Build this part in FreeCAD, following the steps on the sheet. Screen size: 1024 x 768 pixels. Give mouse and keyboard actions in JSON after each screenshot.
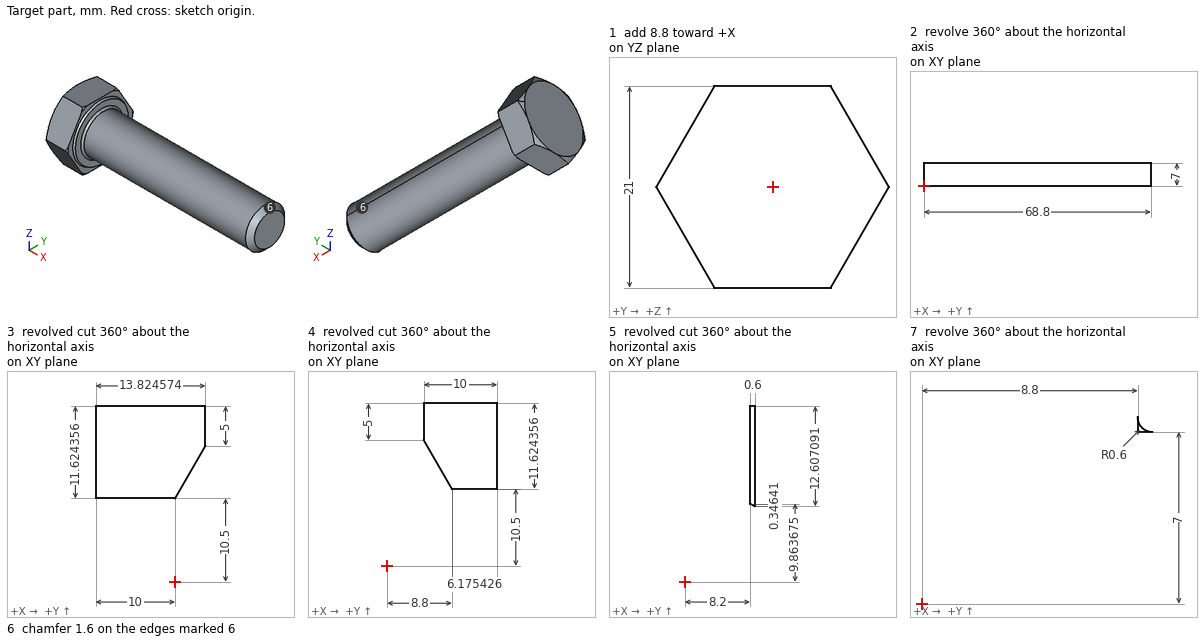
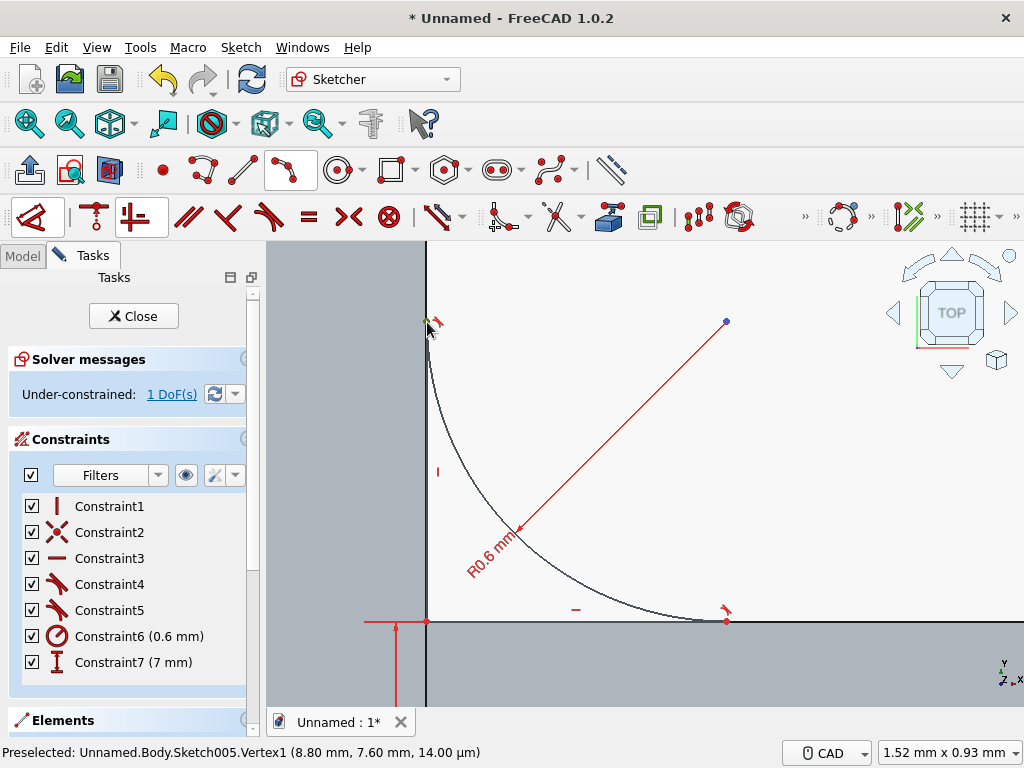
{"action": "key", "text": "l"}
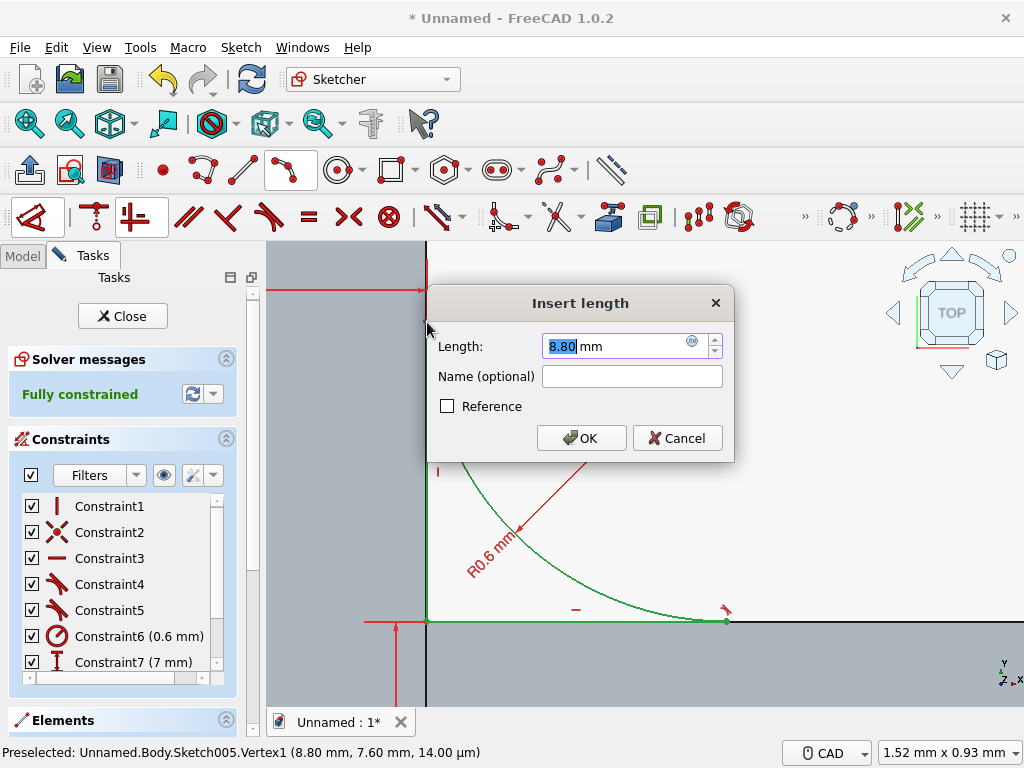
{"action": "type", "text": "8.8"}
{"action": "key", "text": "Return"}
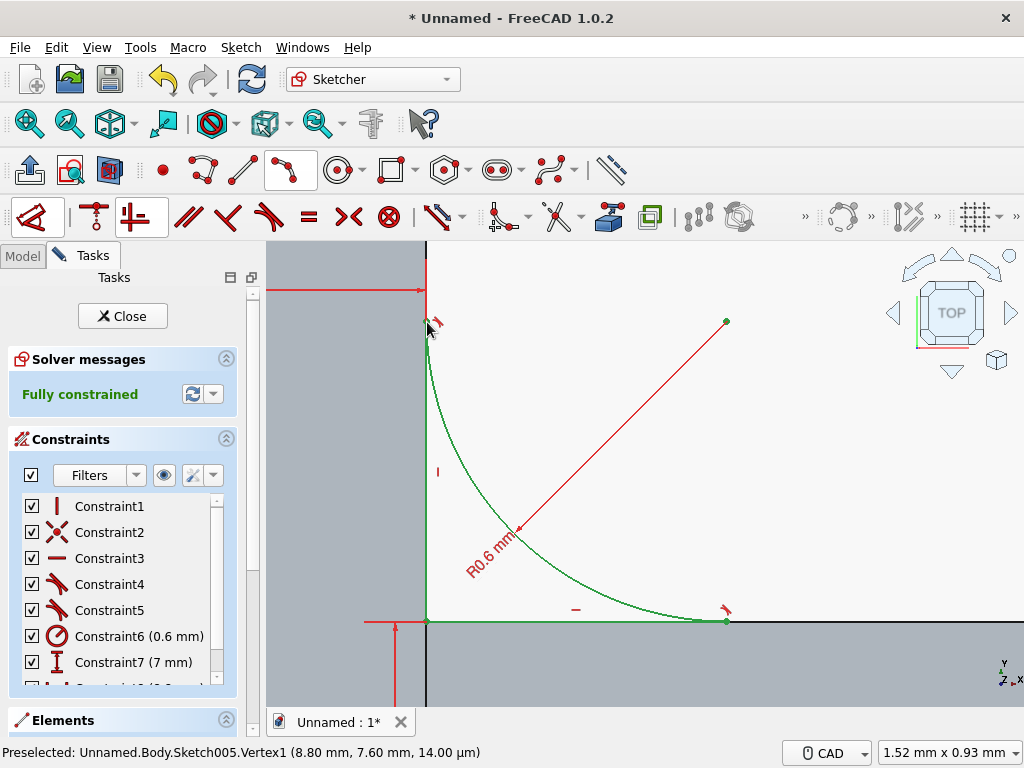
{"action": "left_click", "coordinate": [123, 316]}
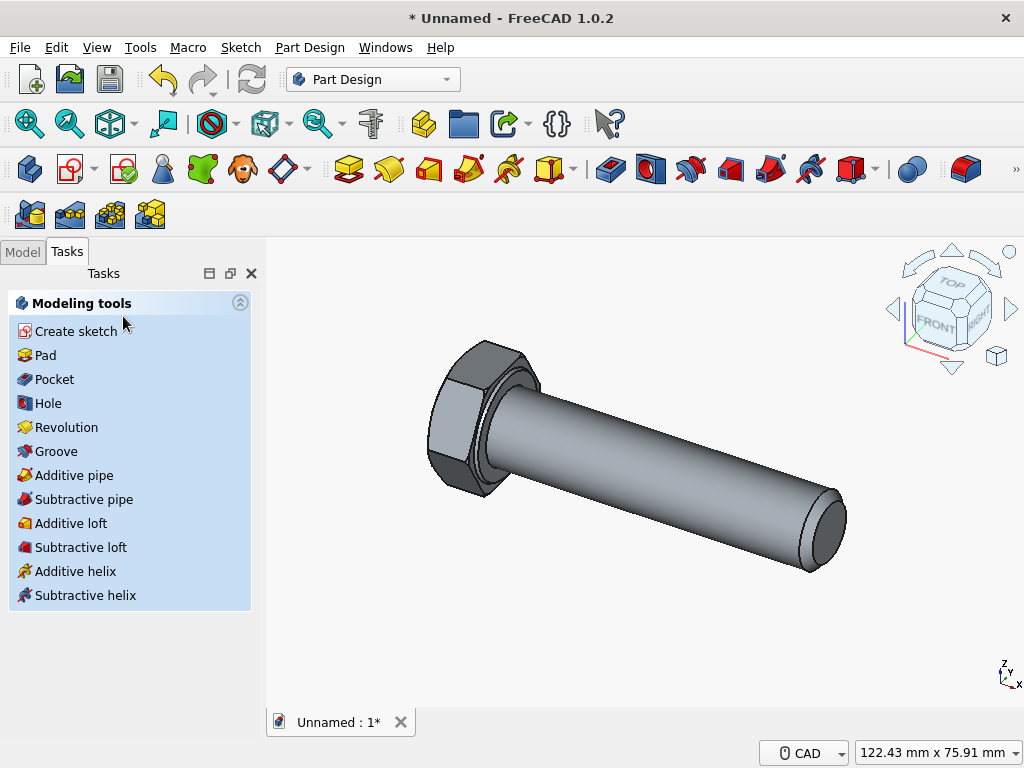
{"action": "left_click", "coordinate": [390, 170]}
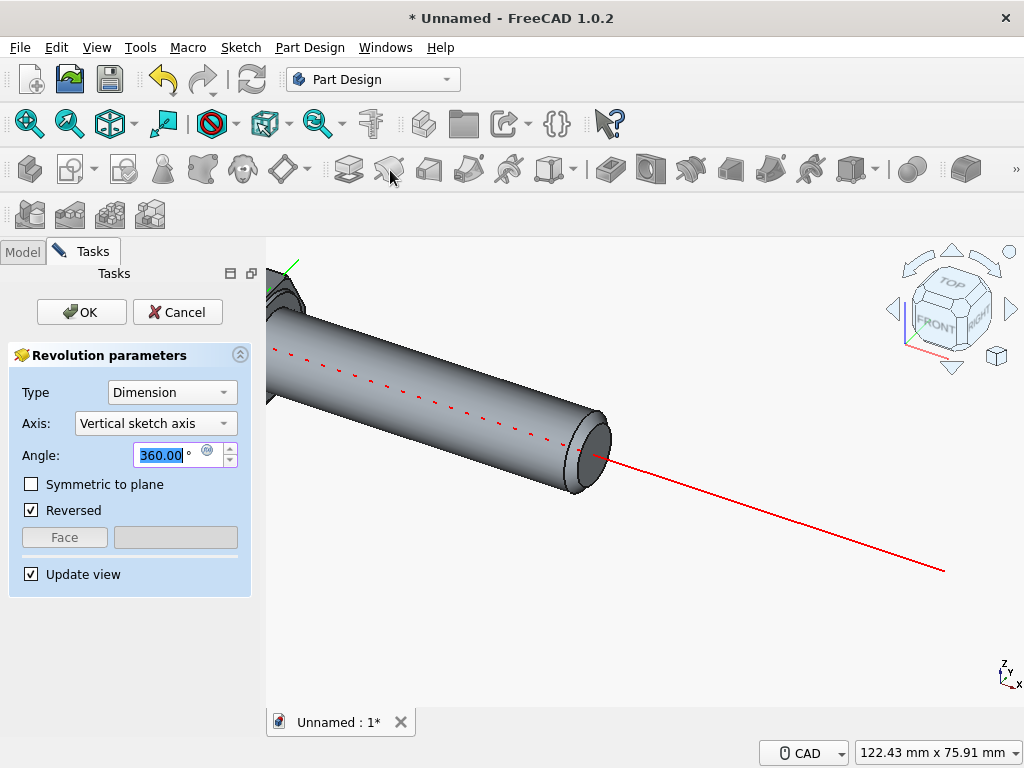
{"action": "left_click", "coordinate": [156, 424]}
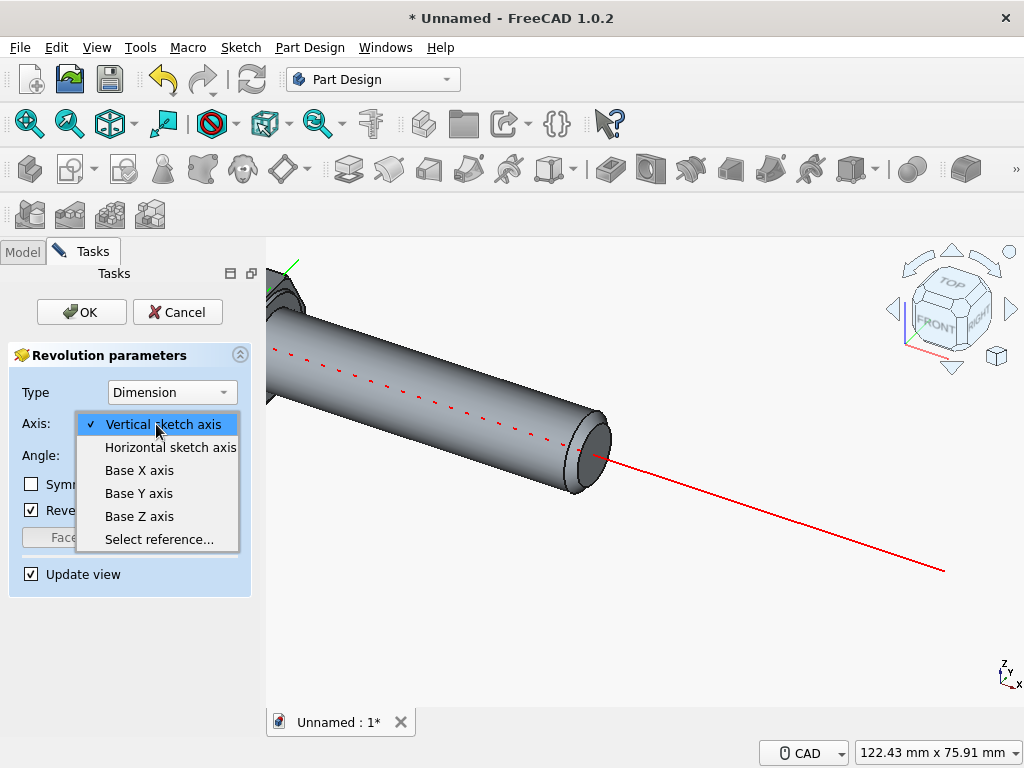
{"action": "left_click", "coordinate": [156, 448]}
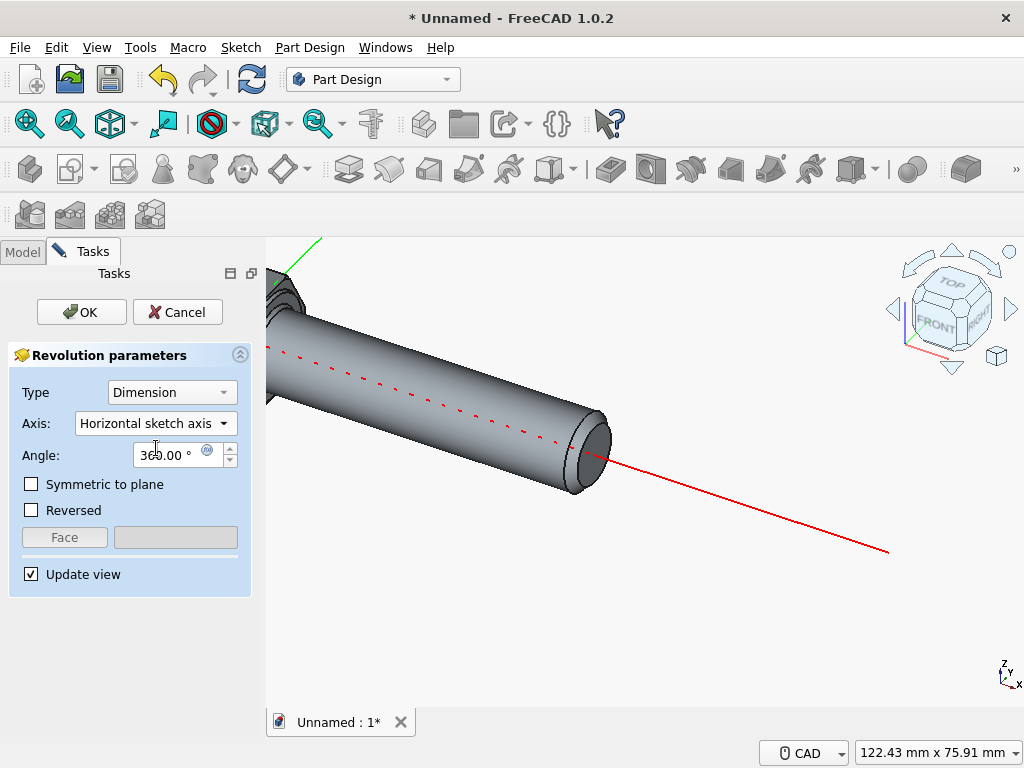
{"action": "left_click", "coordinate": [82, 312]}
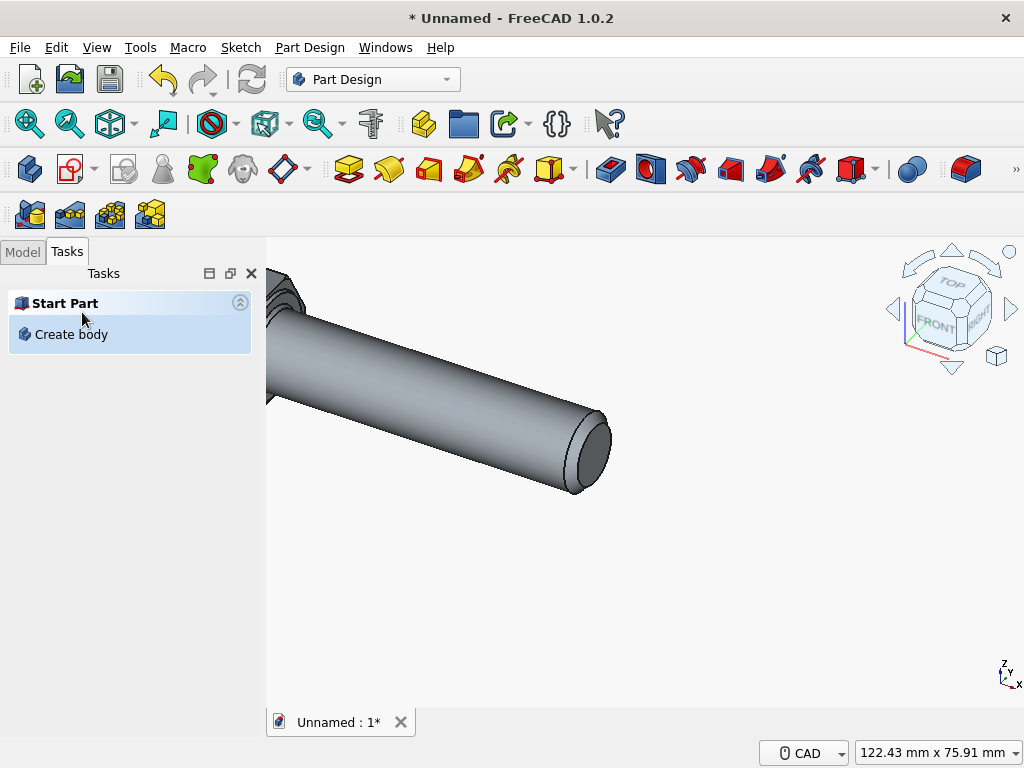
{"action": "key", "text": "0"}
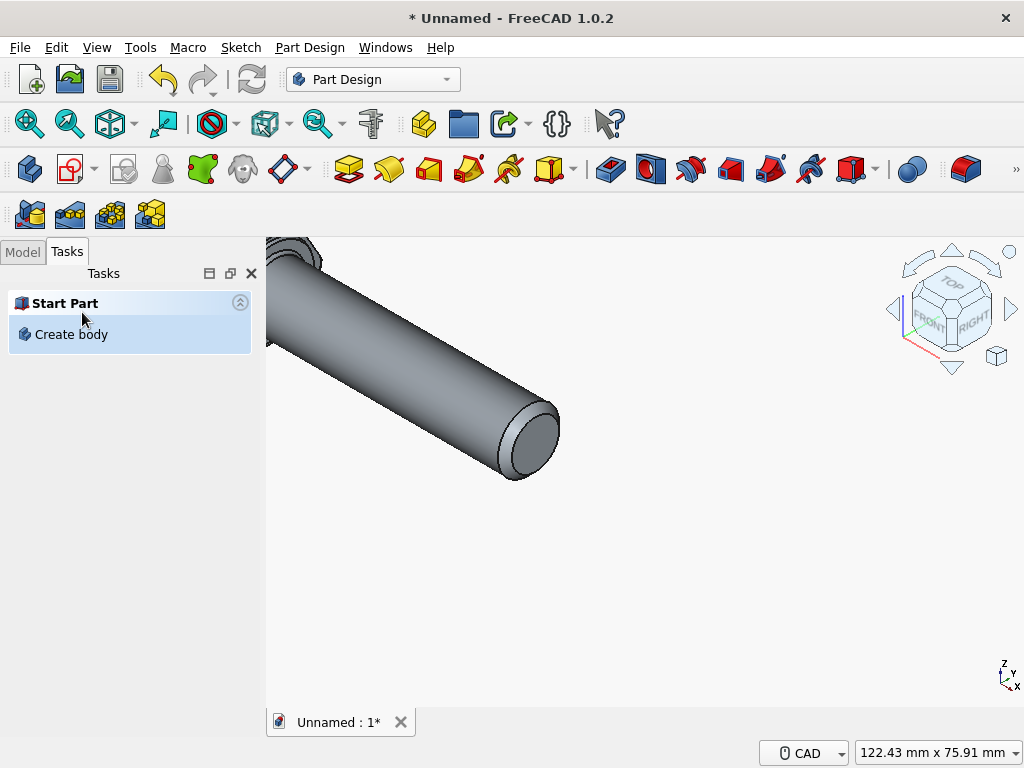
{"action": "left_click", "coordinate": [30, 124]}